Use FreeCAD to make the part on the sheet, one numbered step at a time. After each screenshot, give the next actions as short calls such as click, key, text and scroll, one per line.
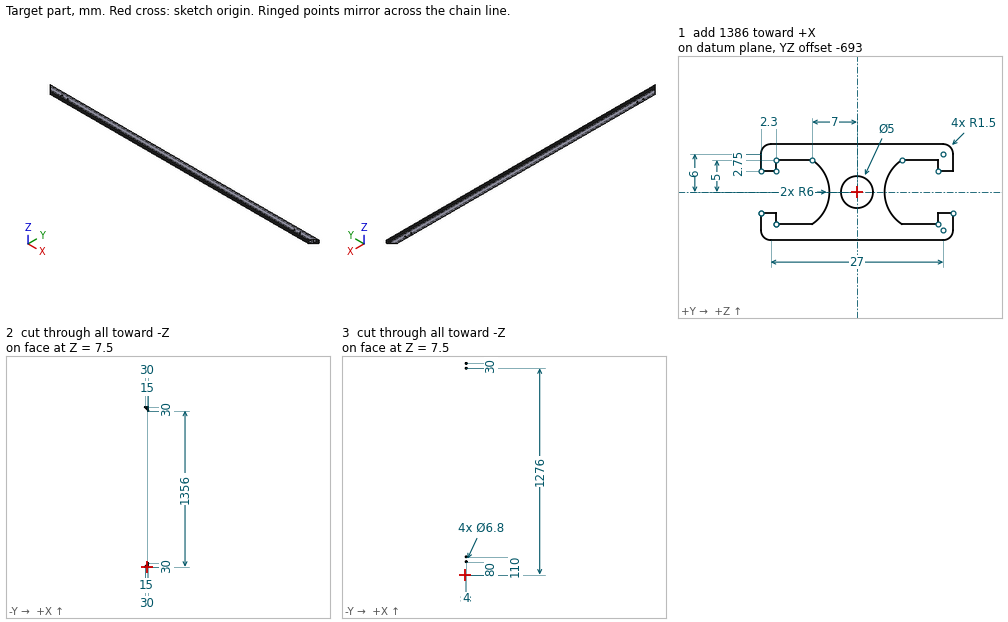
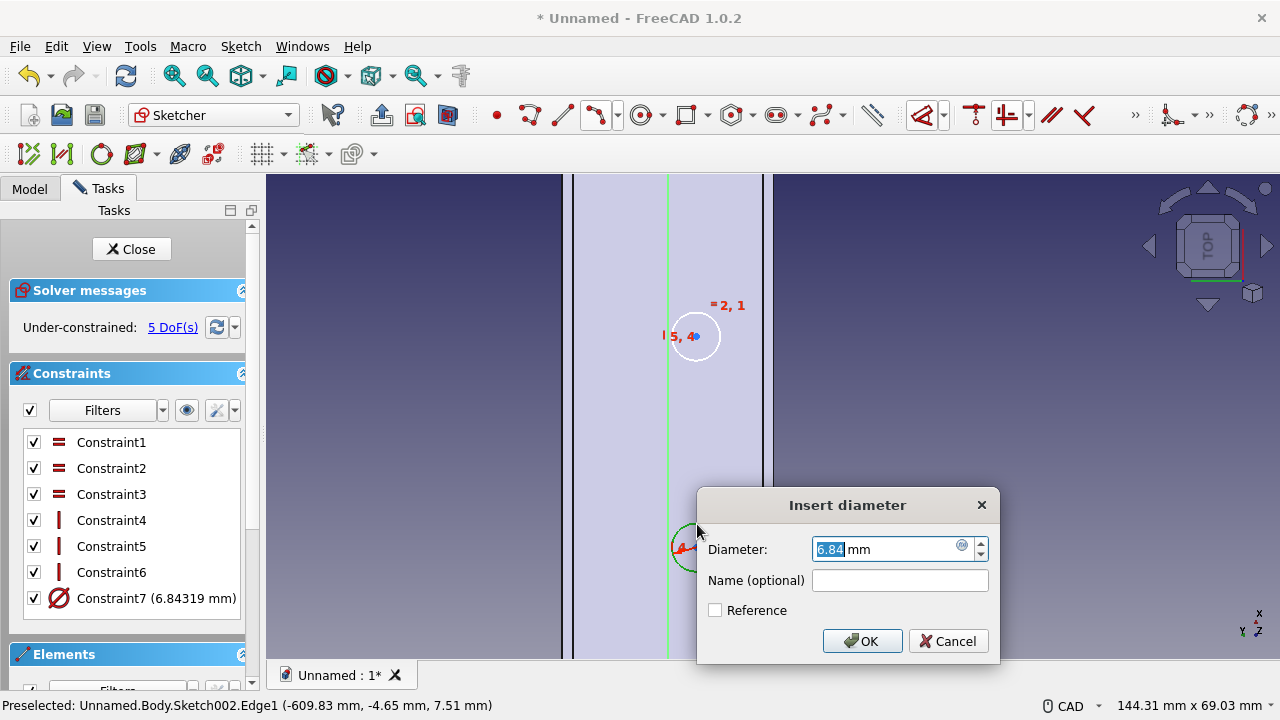
text(6.8)
key(Return)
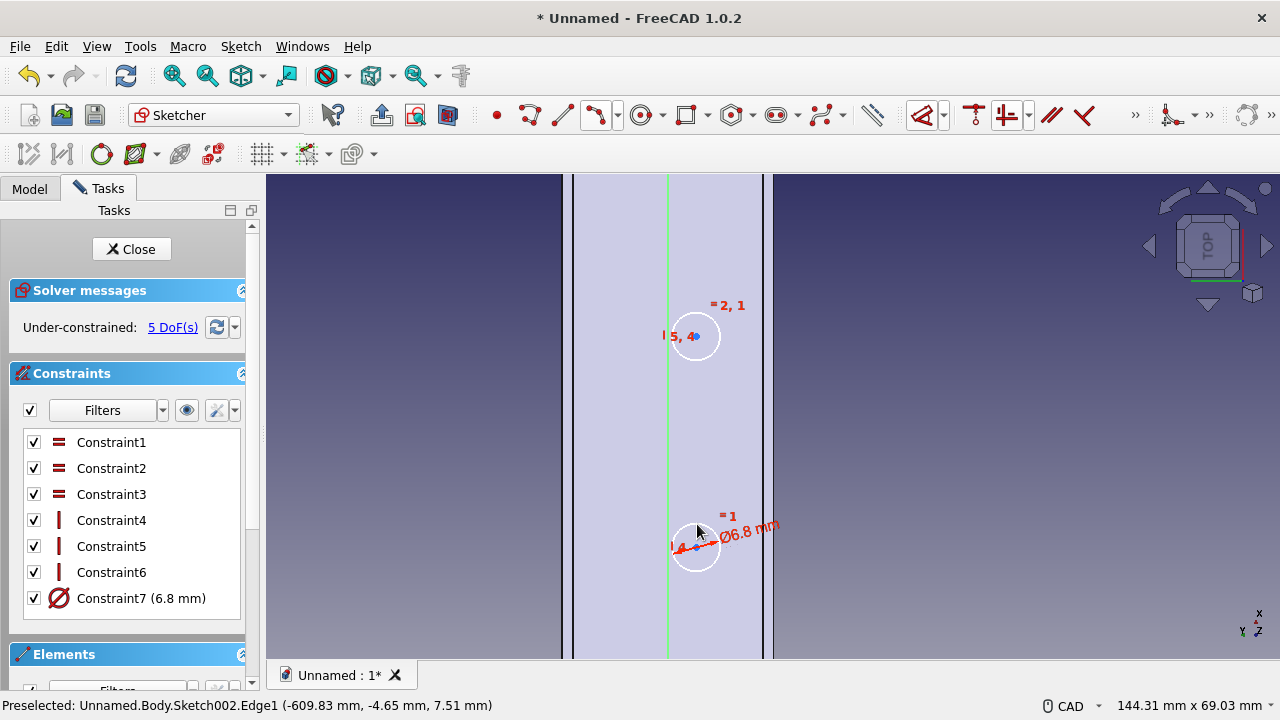
scroll(696, 548, up, 2)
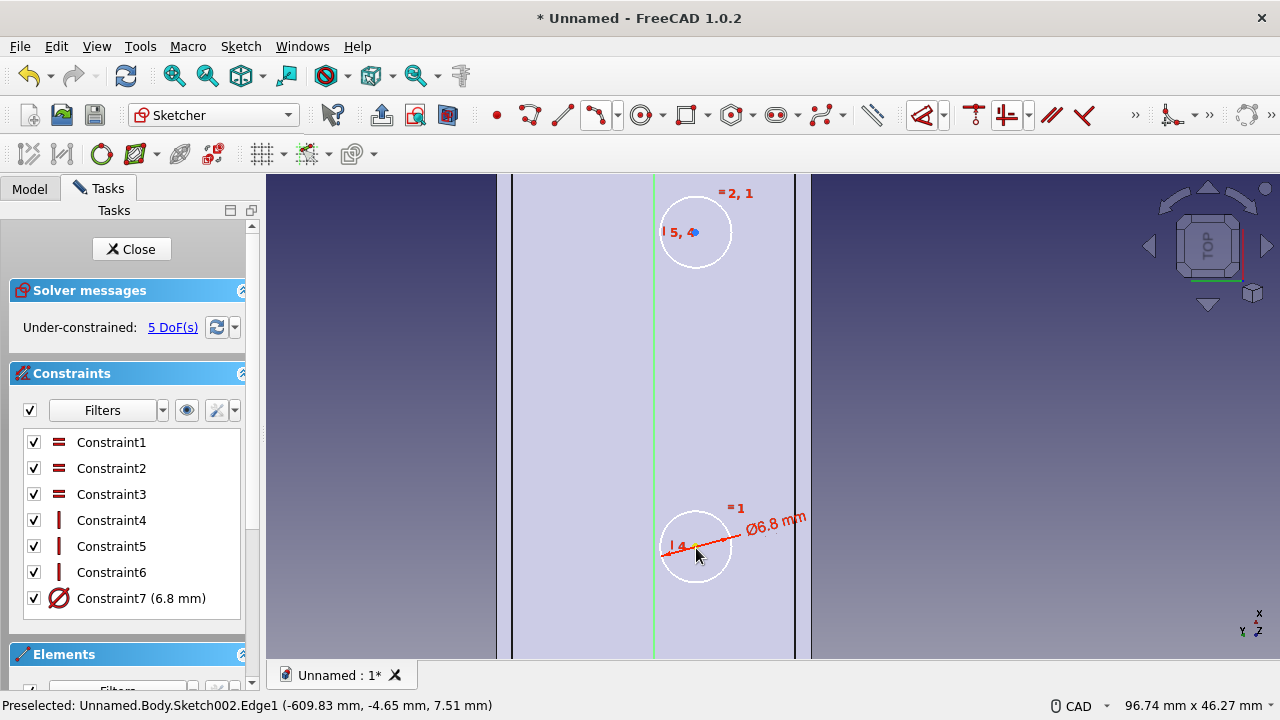
click(696, 547)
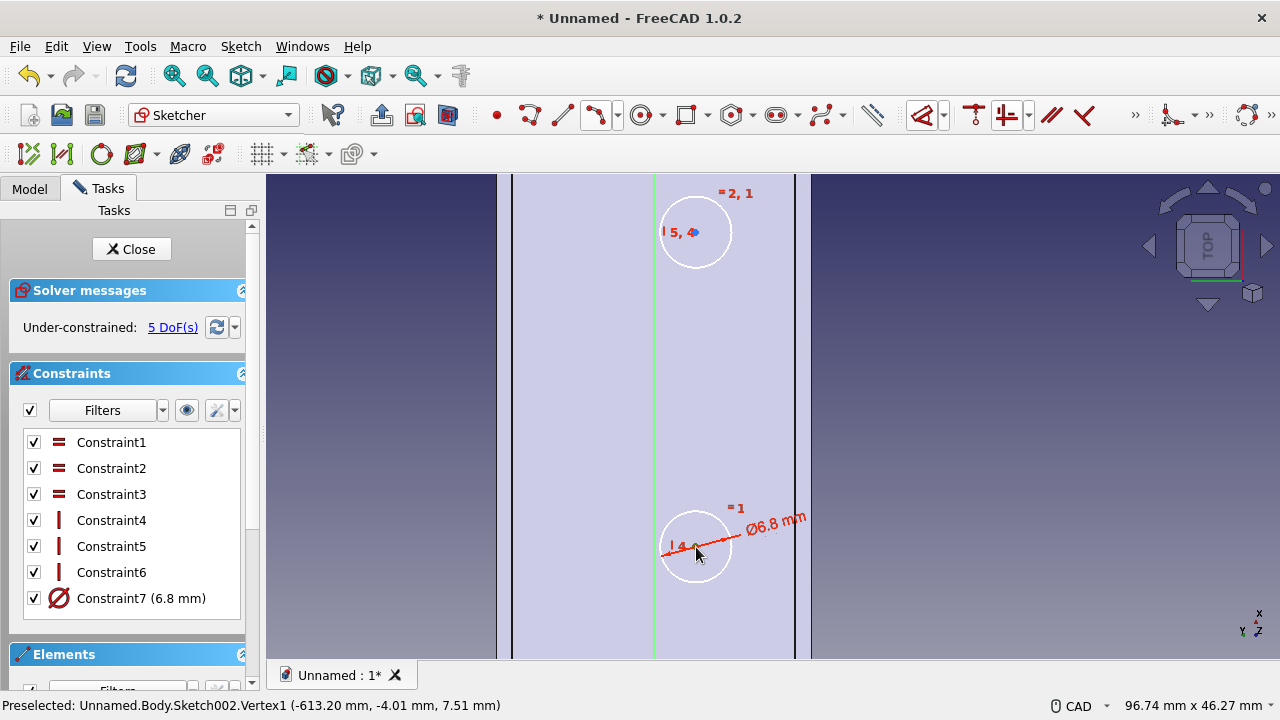
key(l)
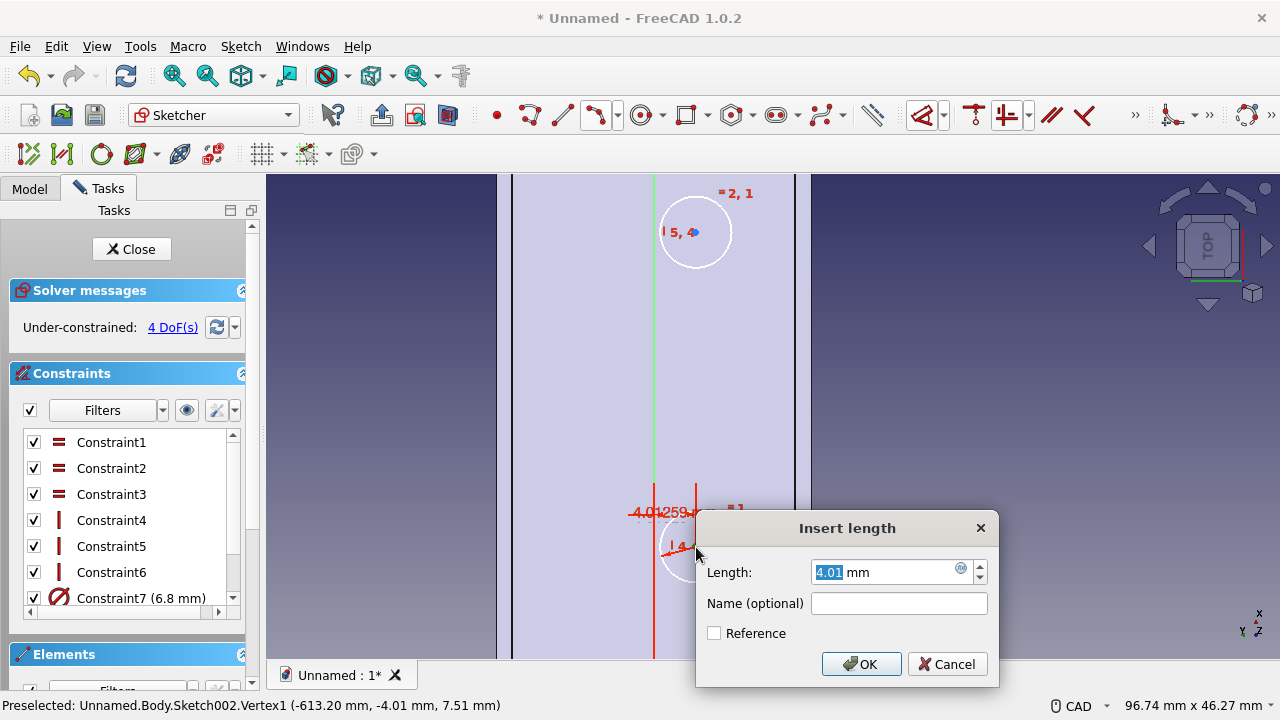
text(4)
key(Return)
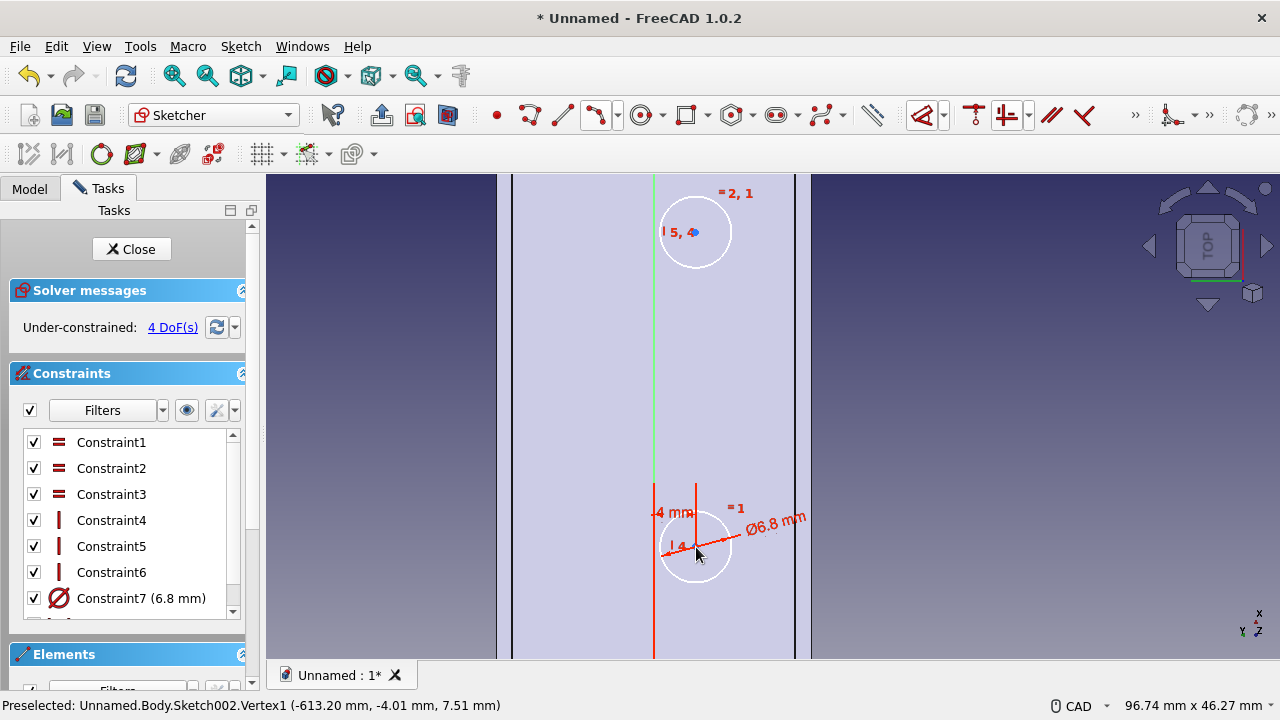
scroll(705, 582, down, 18)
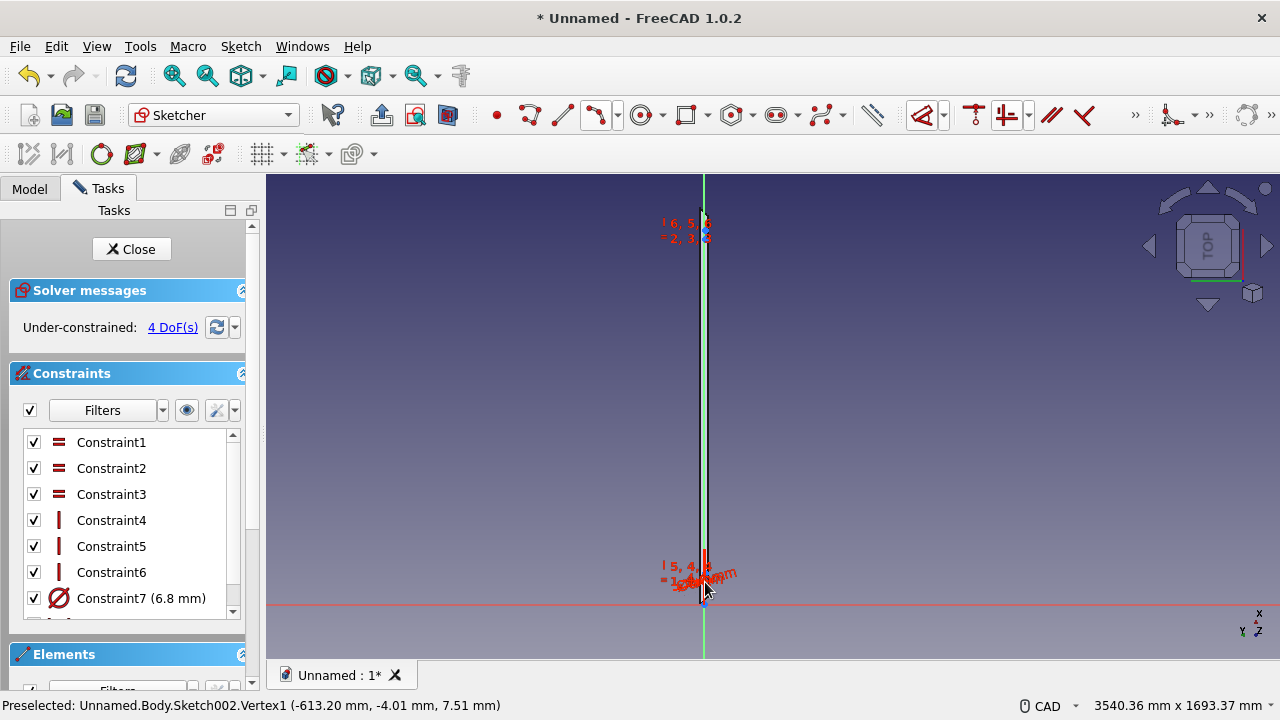
scroll(705, 582, up, 3)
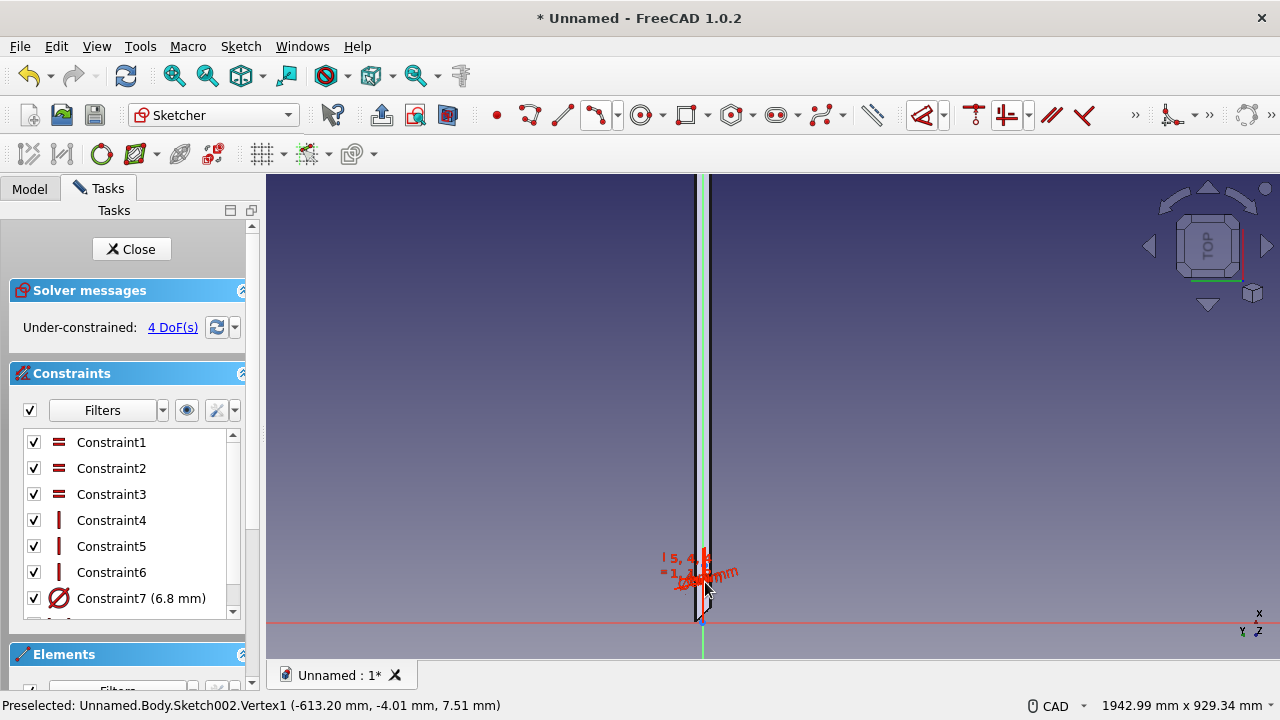
click(705, 581)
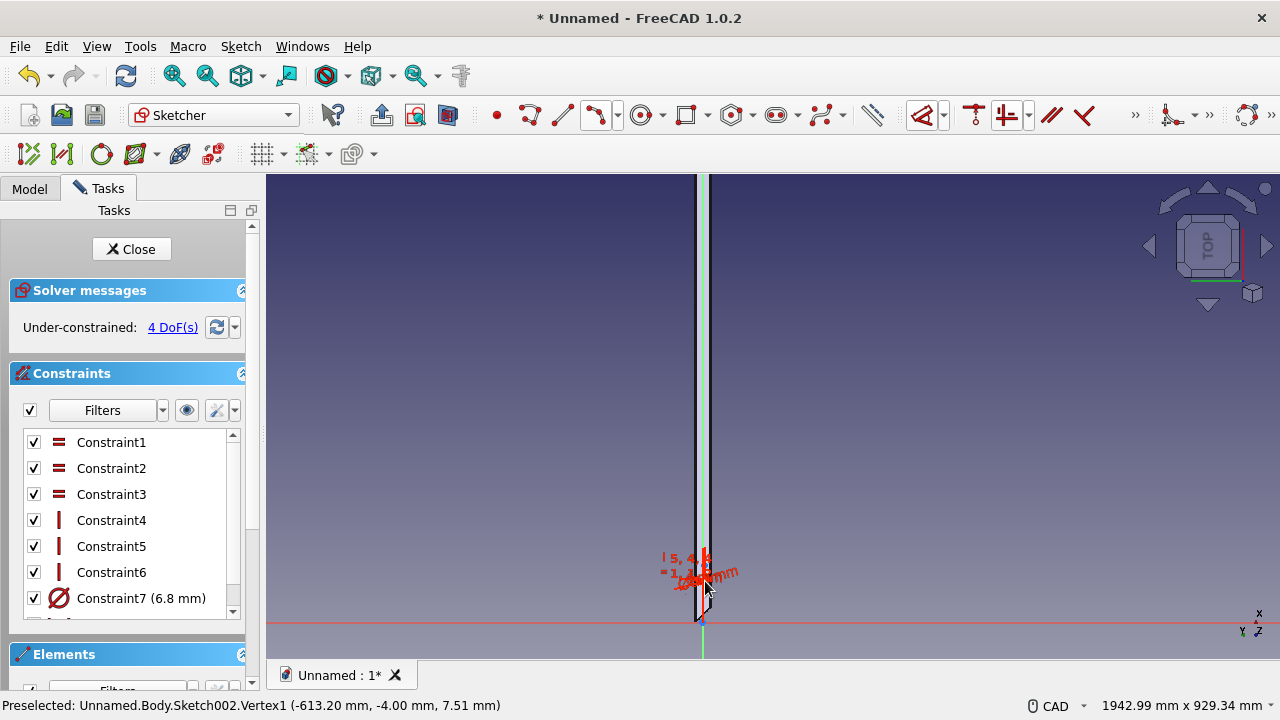
key(i)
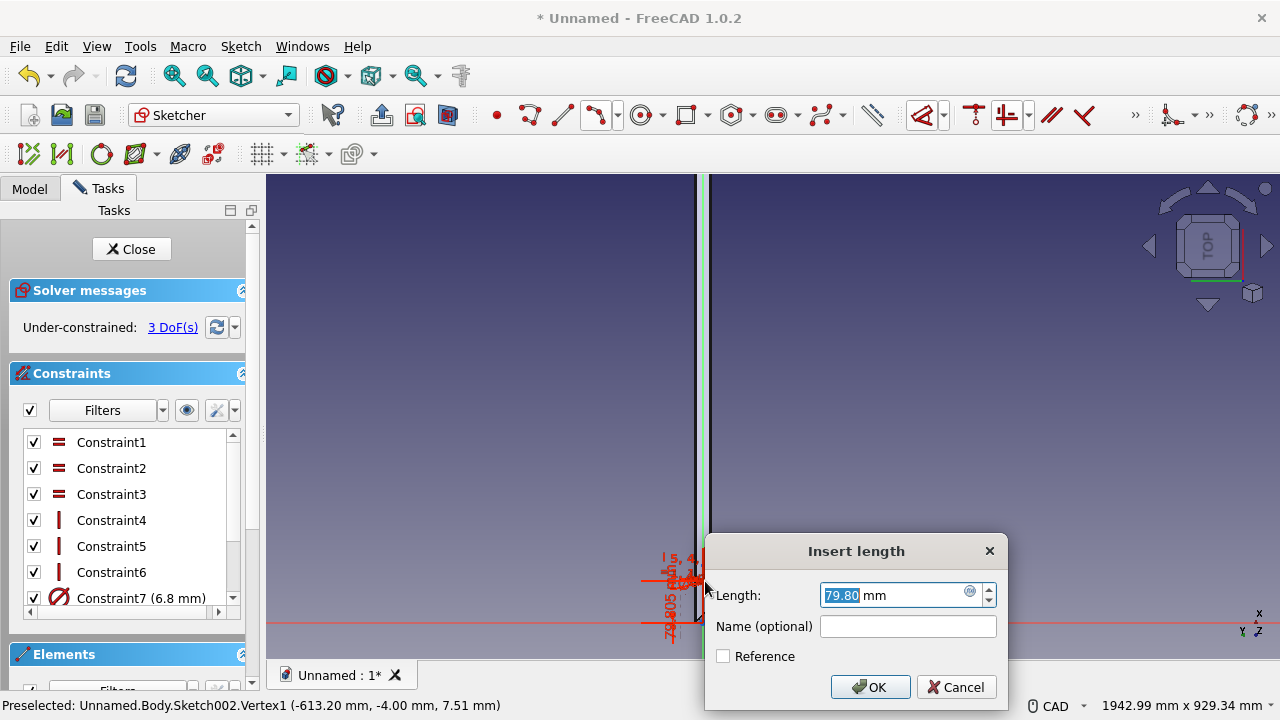
text(80)
key(Return)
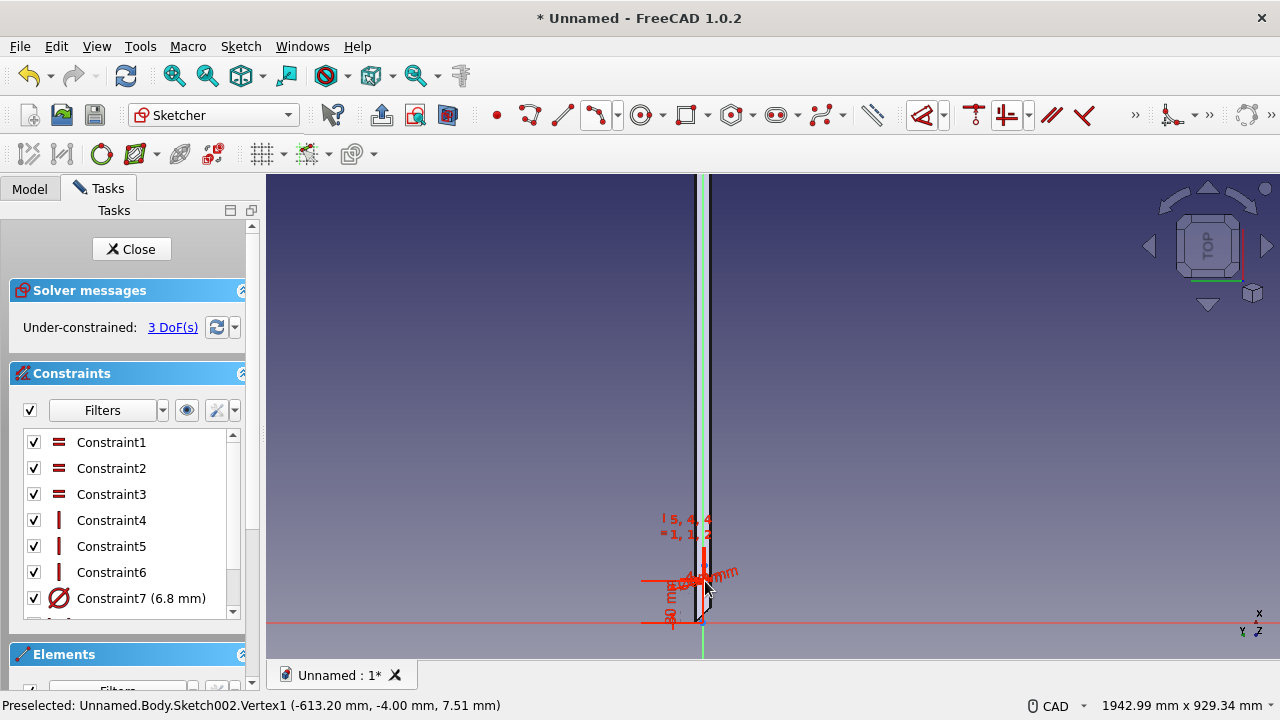
click(705, 565)